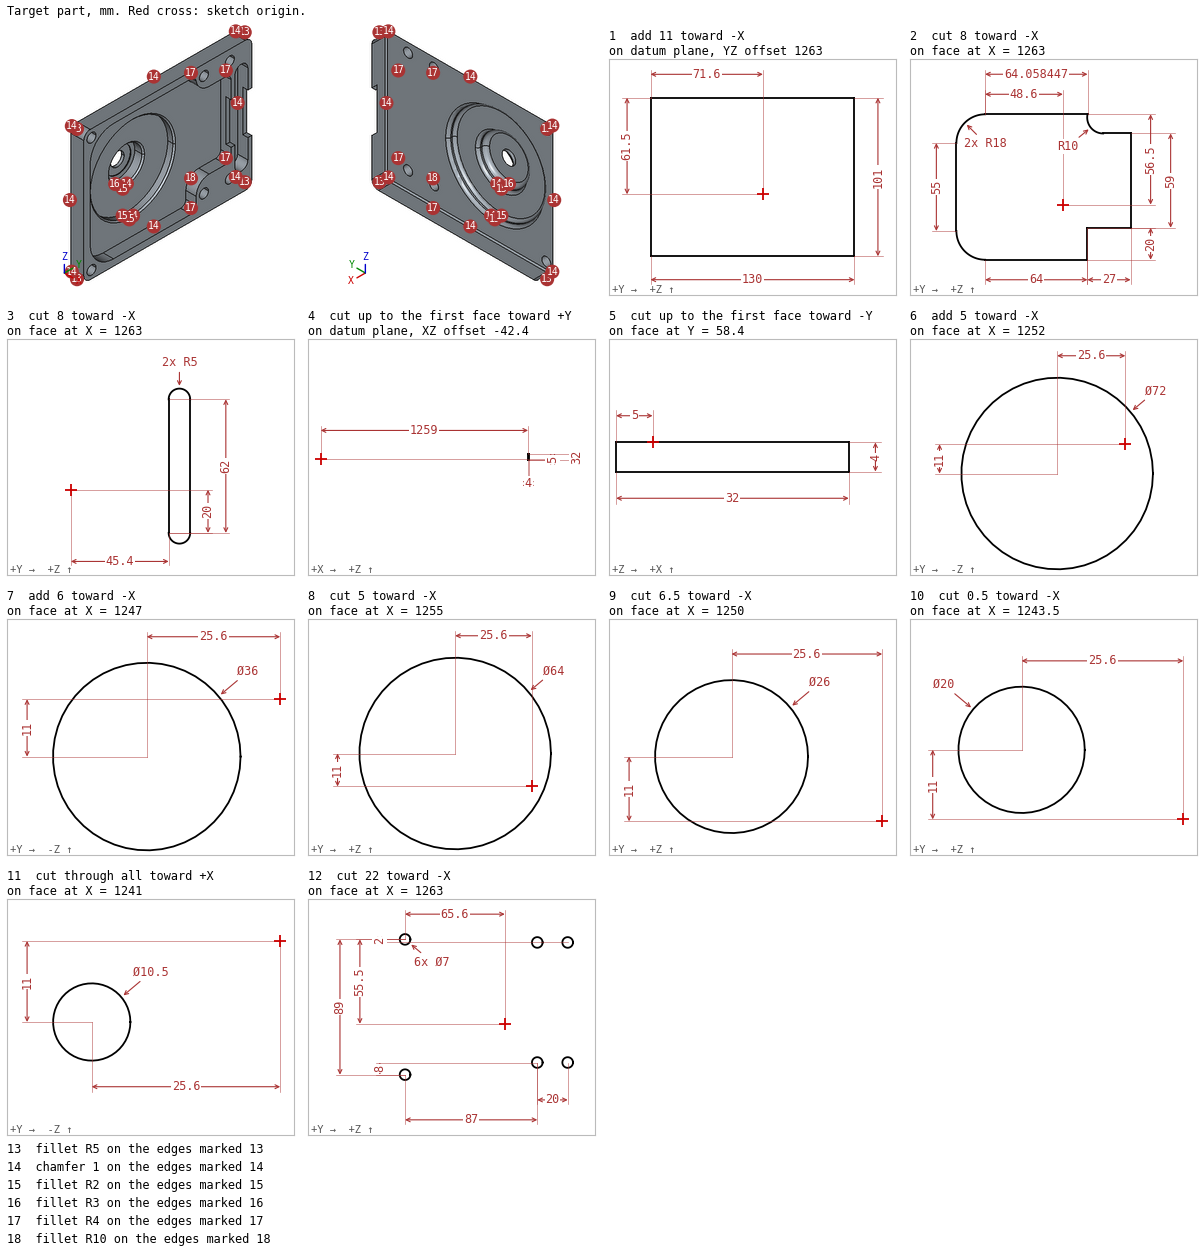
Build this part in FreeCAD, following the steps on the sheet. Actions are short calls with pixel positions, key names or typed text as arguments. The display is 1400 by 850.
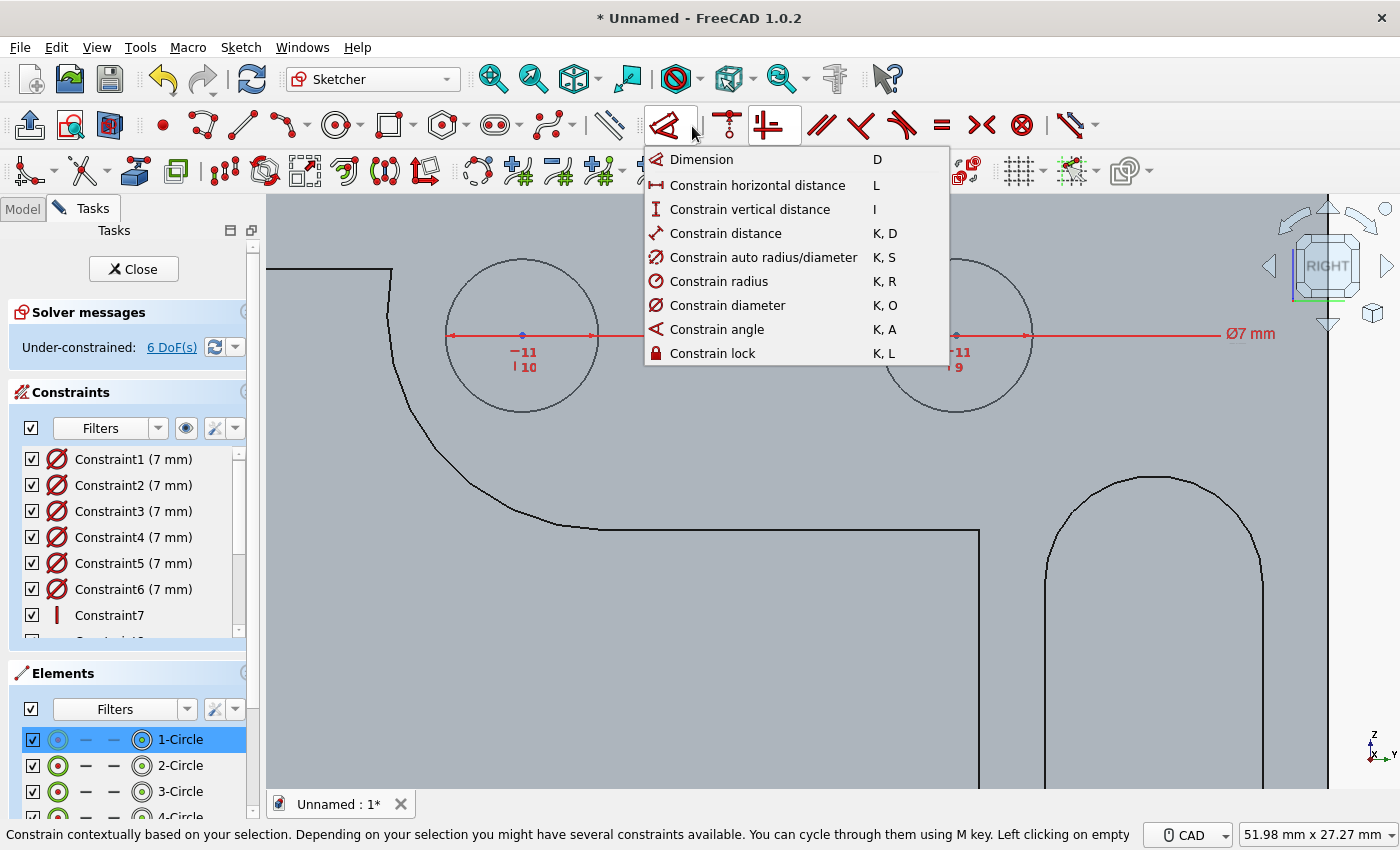
click(797, 209)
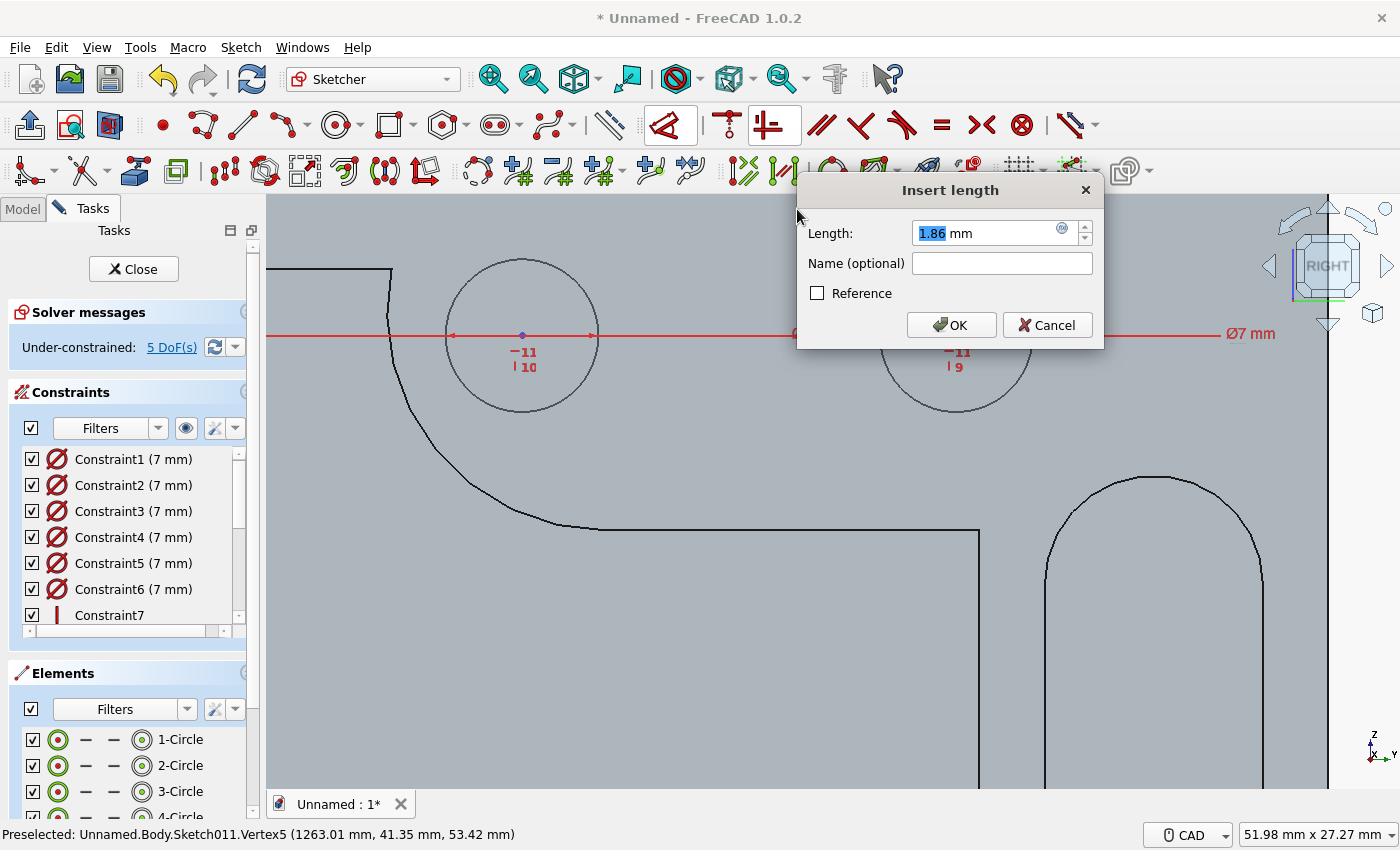
text(2)
key(Return)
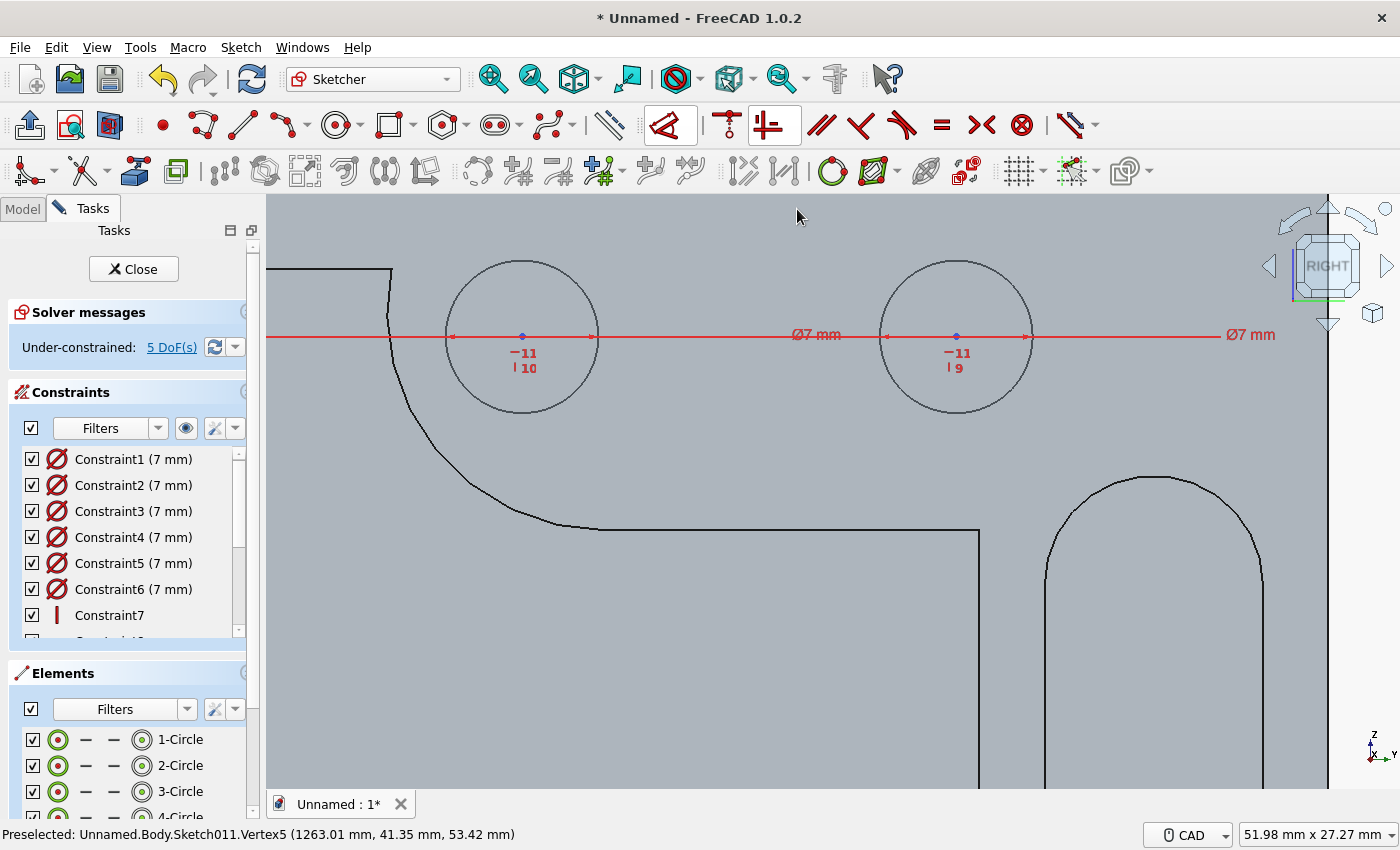
scroll(957, 339, down, 9)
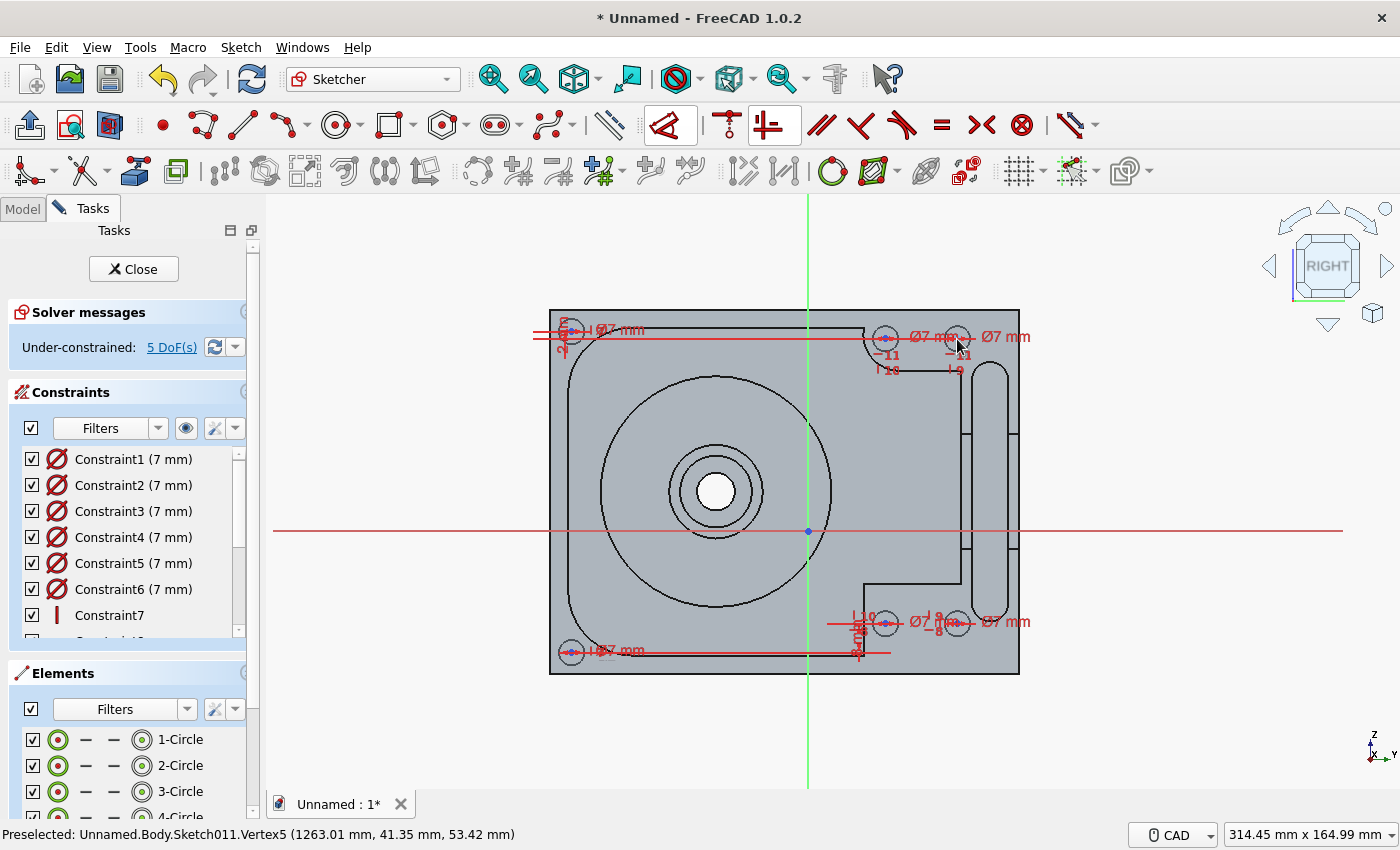
click(572, 332)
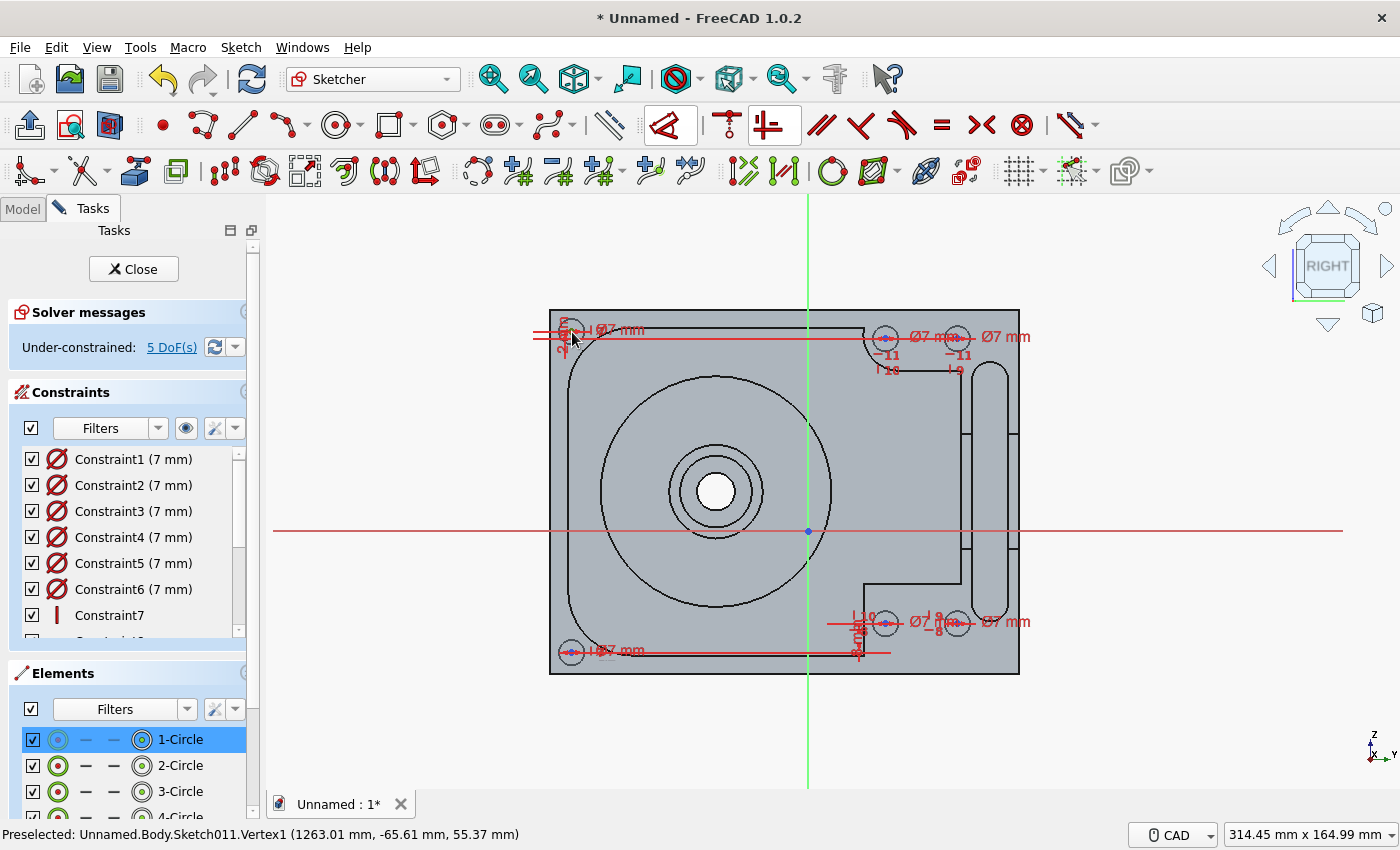
click(572, 653)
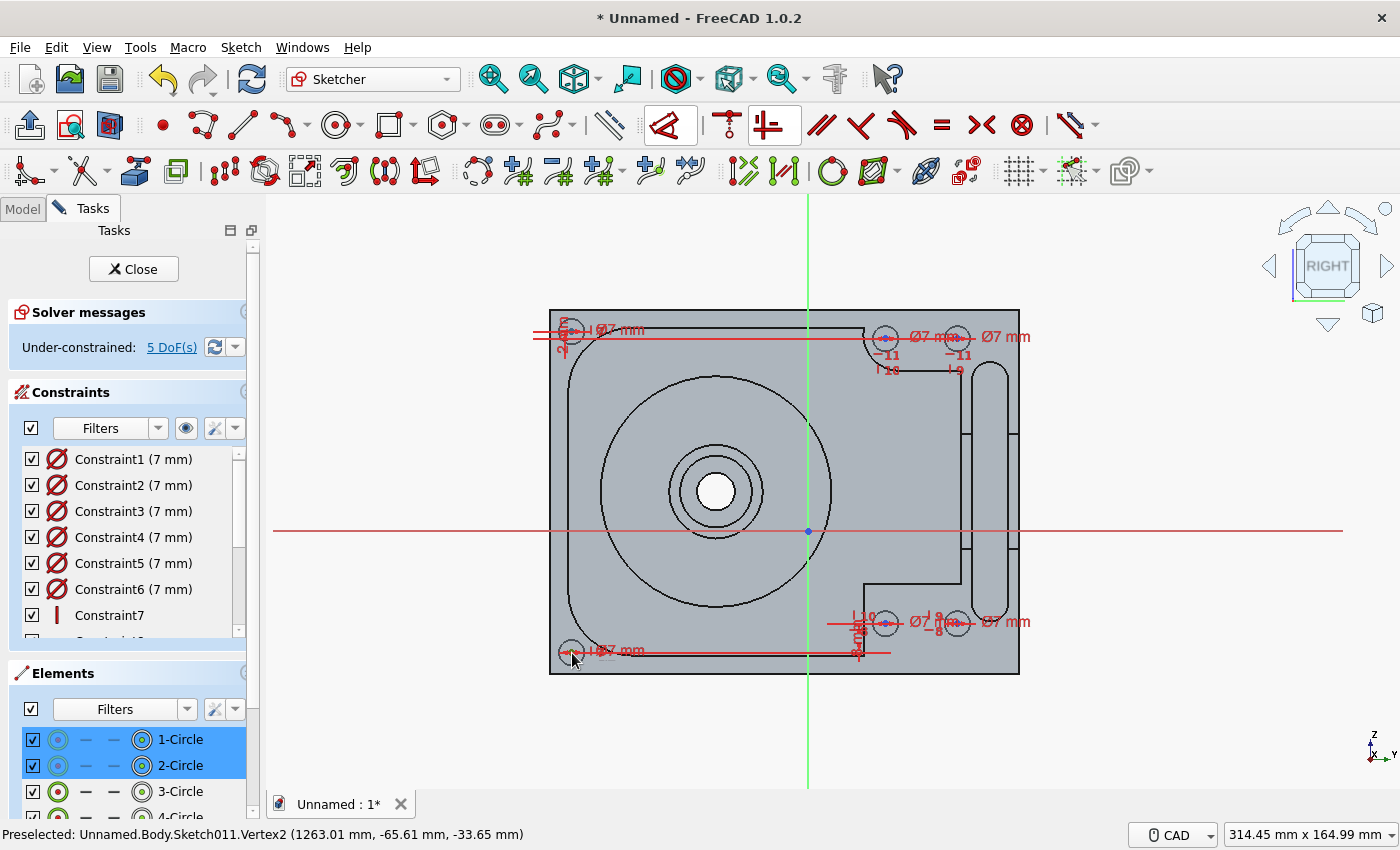
key(i)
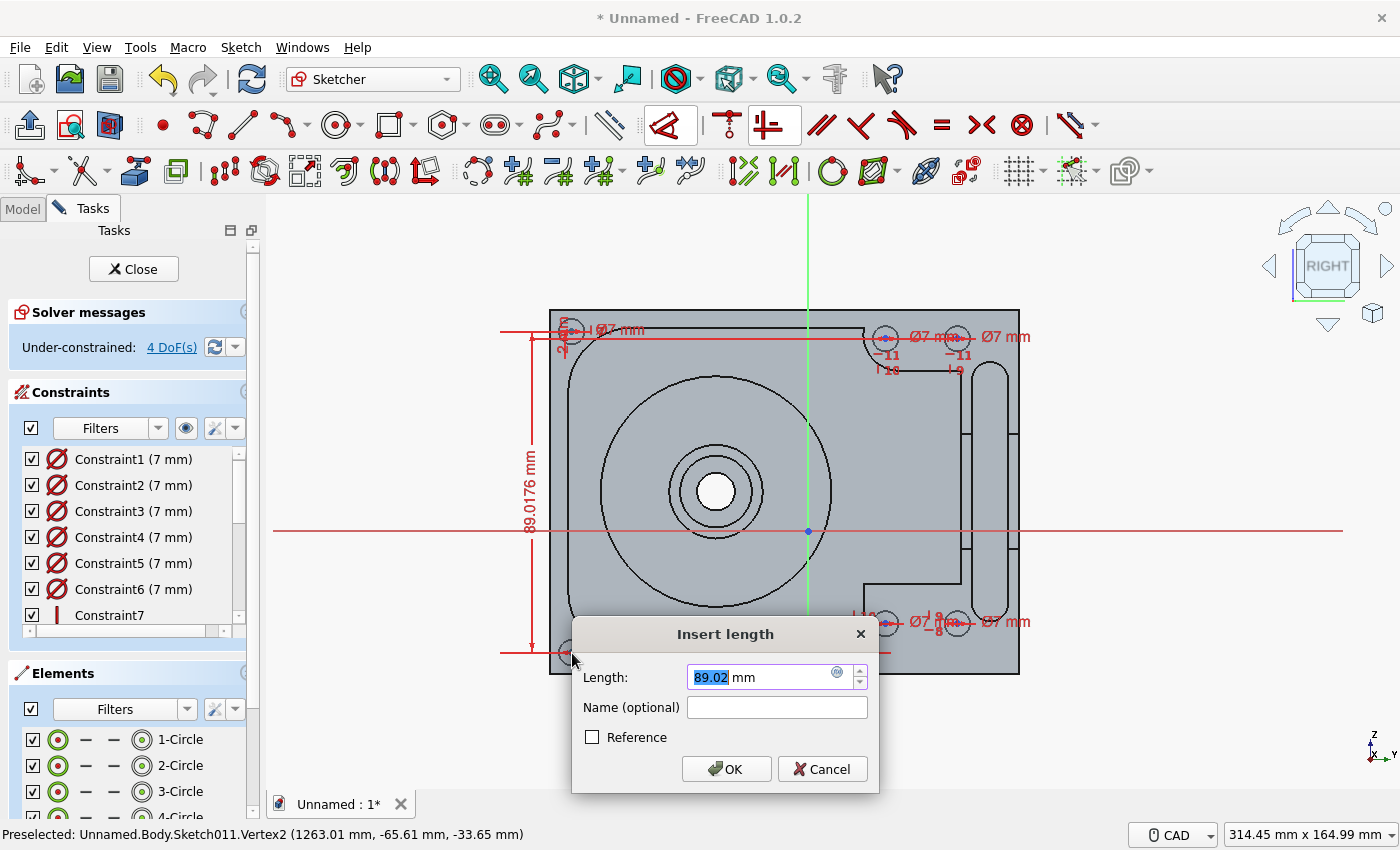
text(89)
key(Return)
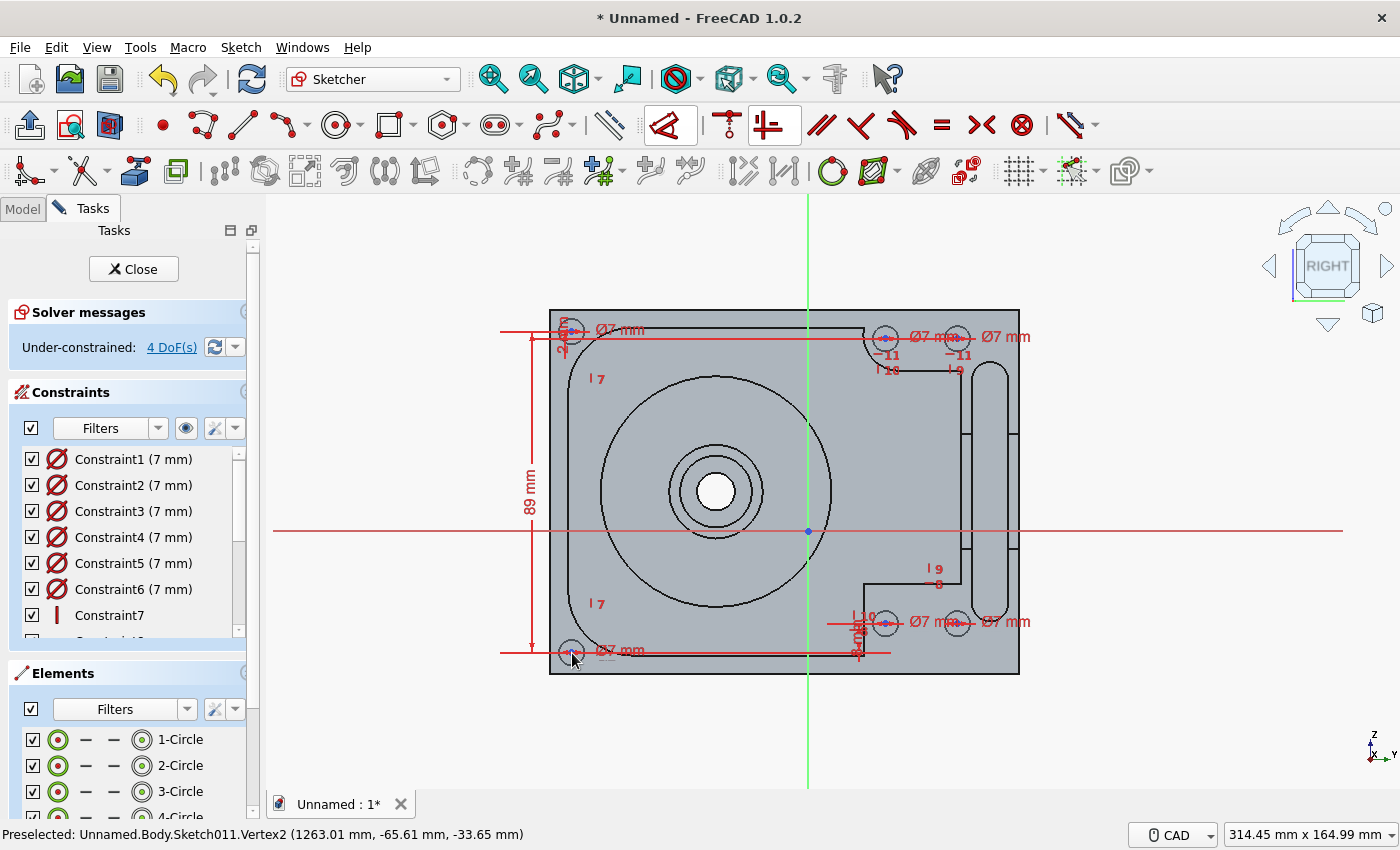
click(572, 653)